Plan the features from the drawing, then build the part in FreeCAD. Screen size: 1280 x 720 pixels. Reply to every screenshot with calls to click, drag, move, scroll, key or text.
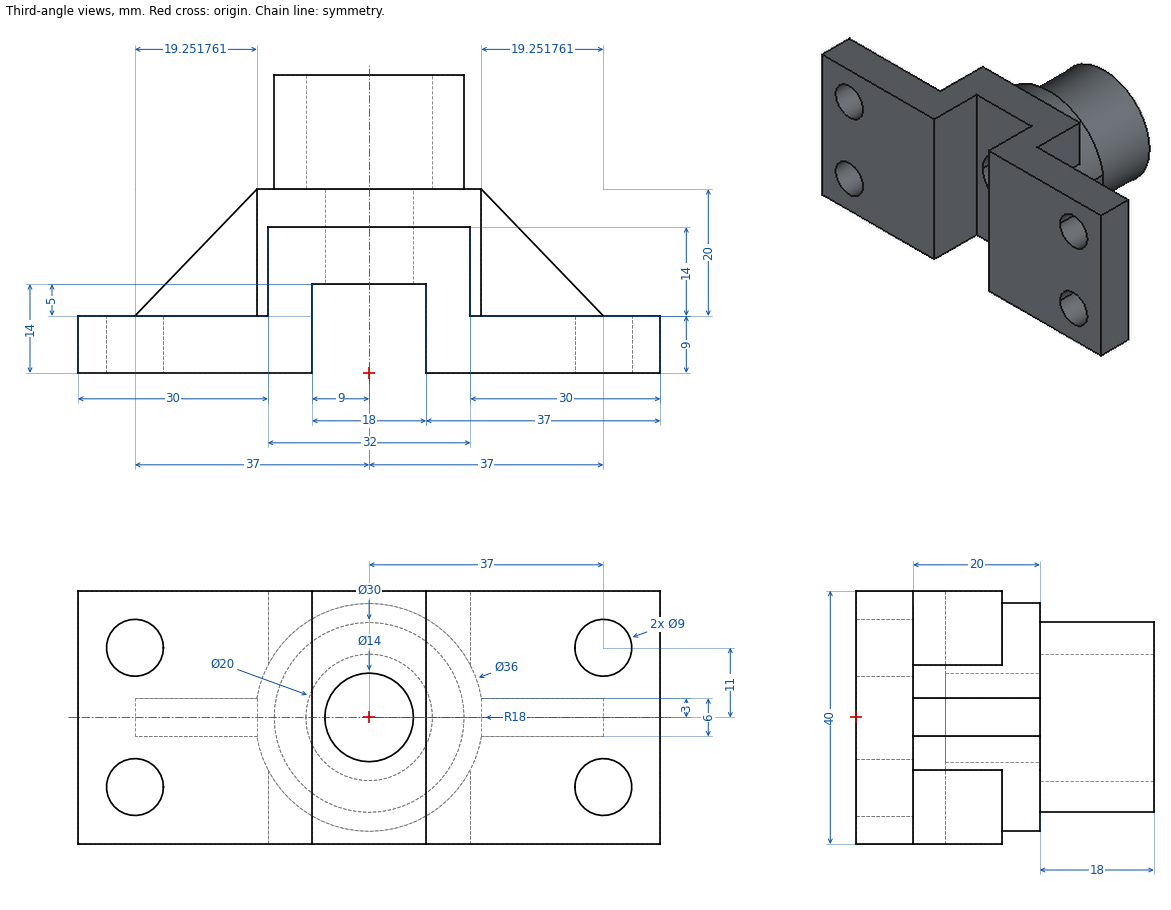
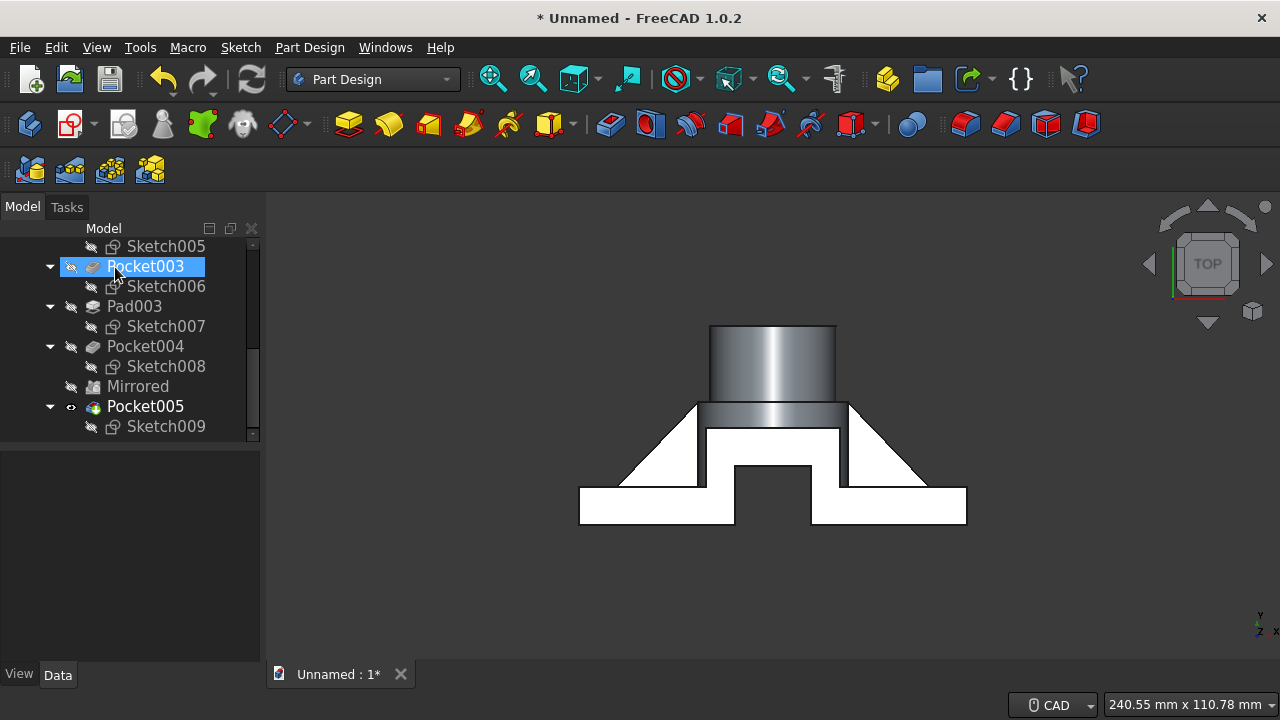
key(0)